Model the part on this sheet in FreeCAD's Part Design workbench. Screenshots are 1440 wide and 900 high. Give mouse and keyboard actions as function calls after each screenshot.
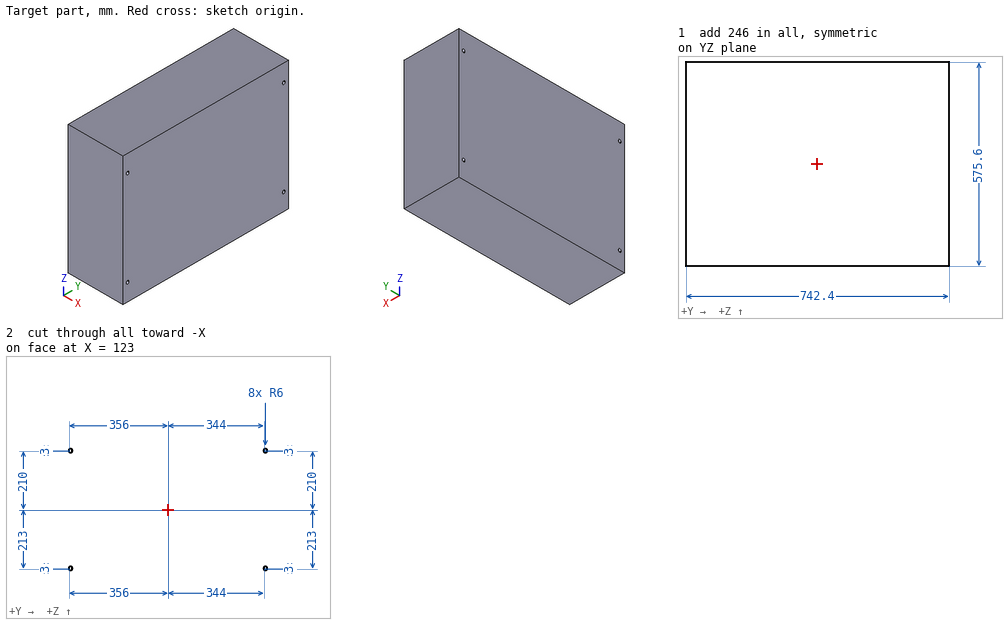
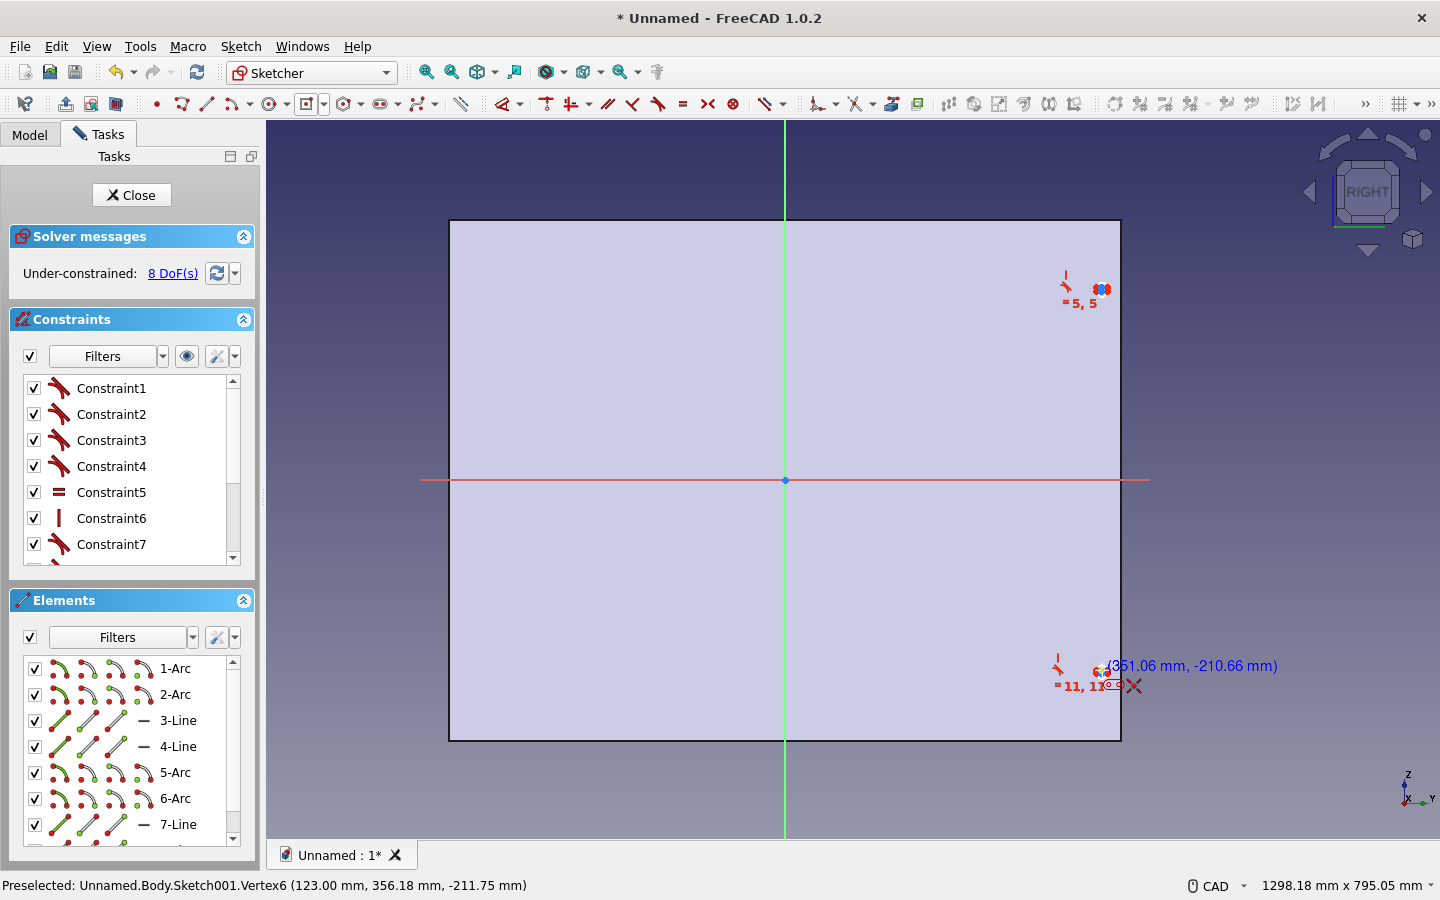
scroll(469, 673, up, 8)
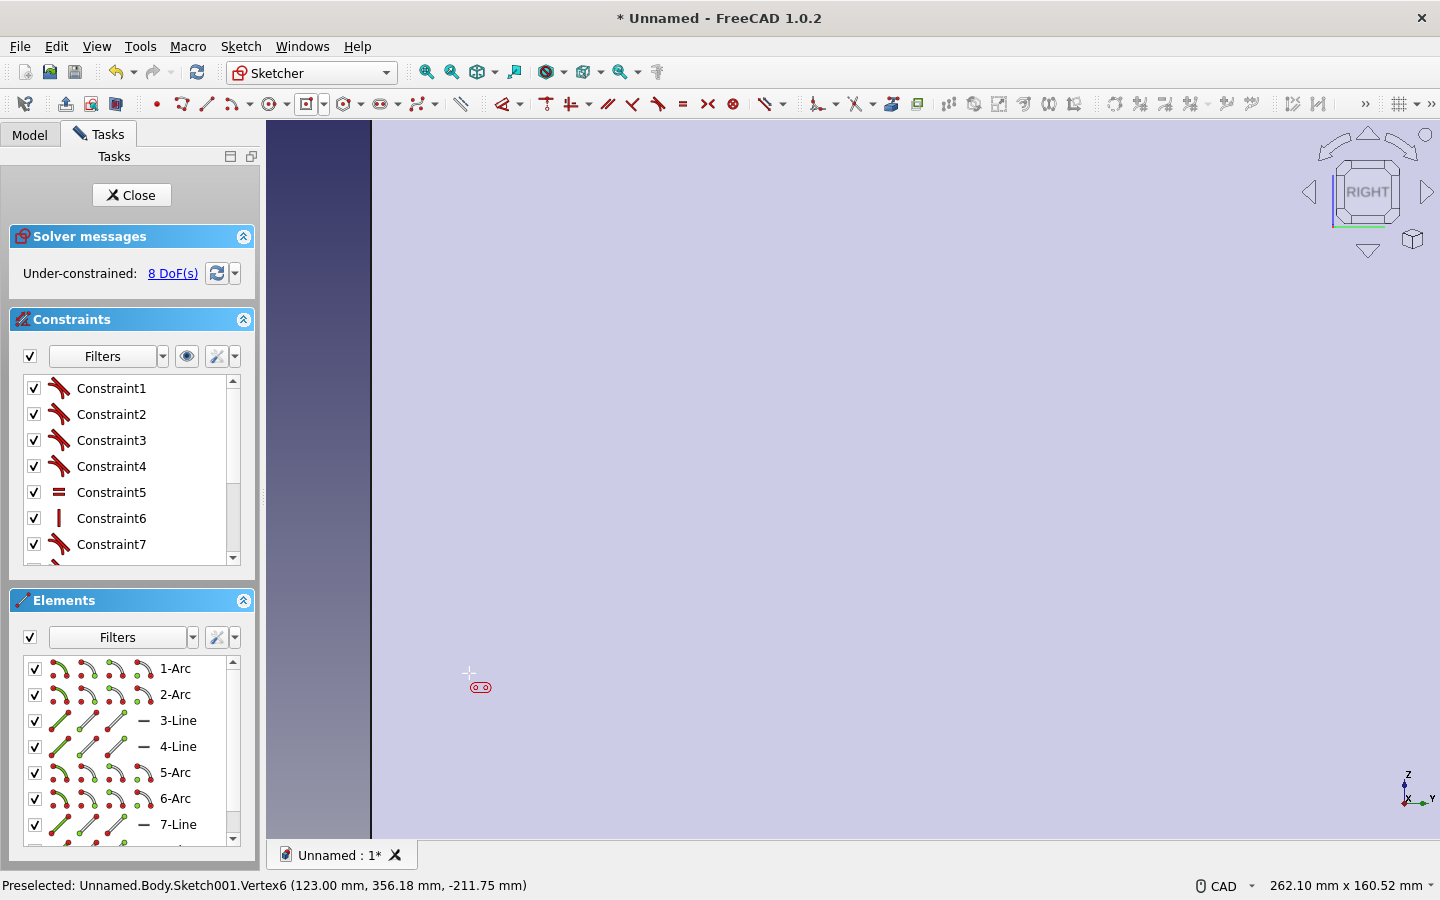
scroll(468, 673, down, 8)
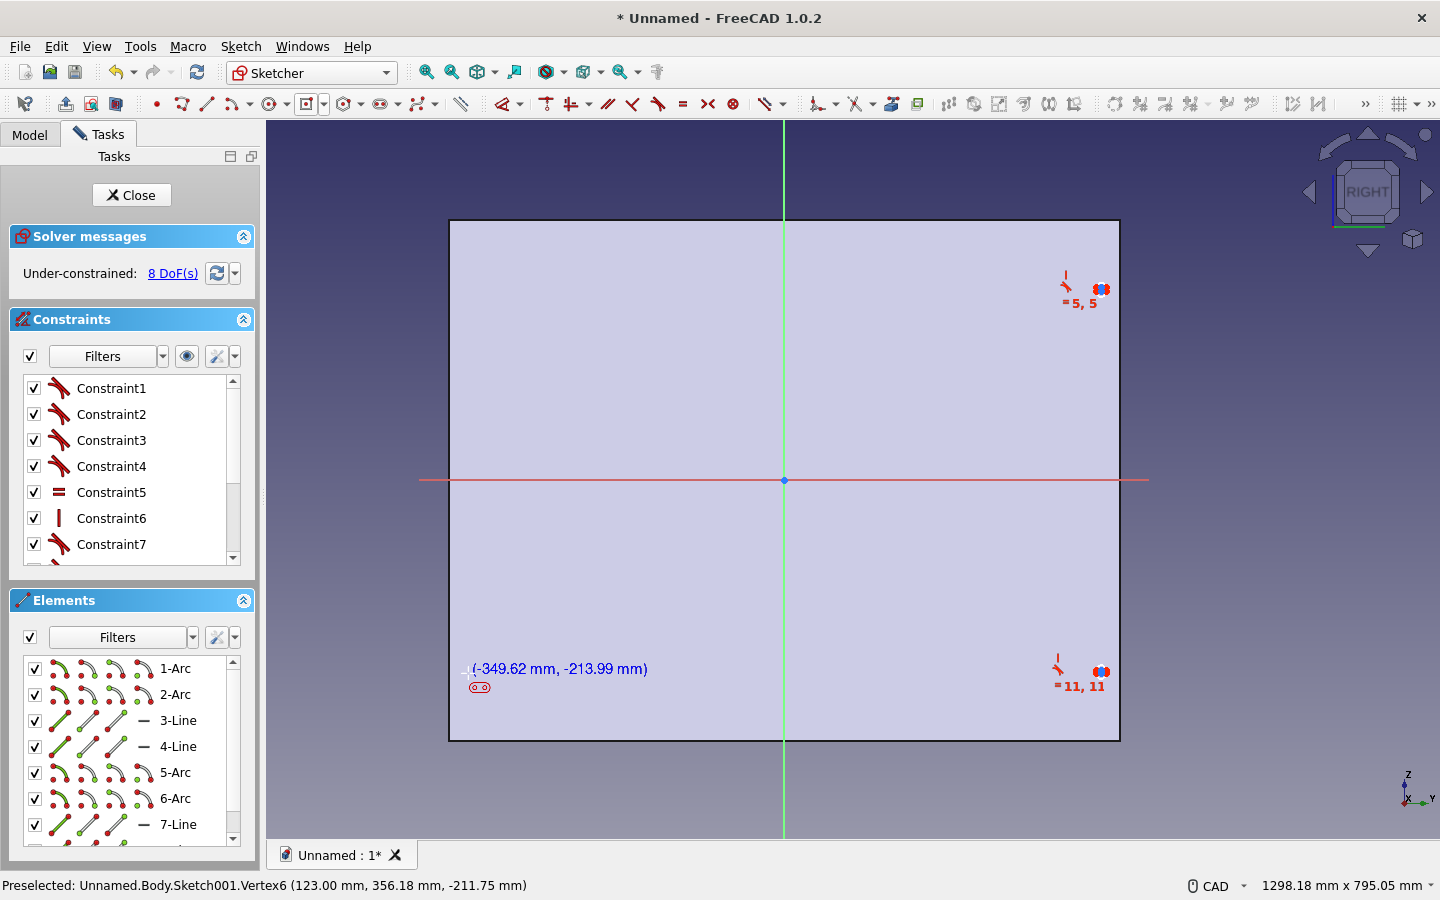
click(468, 673)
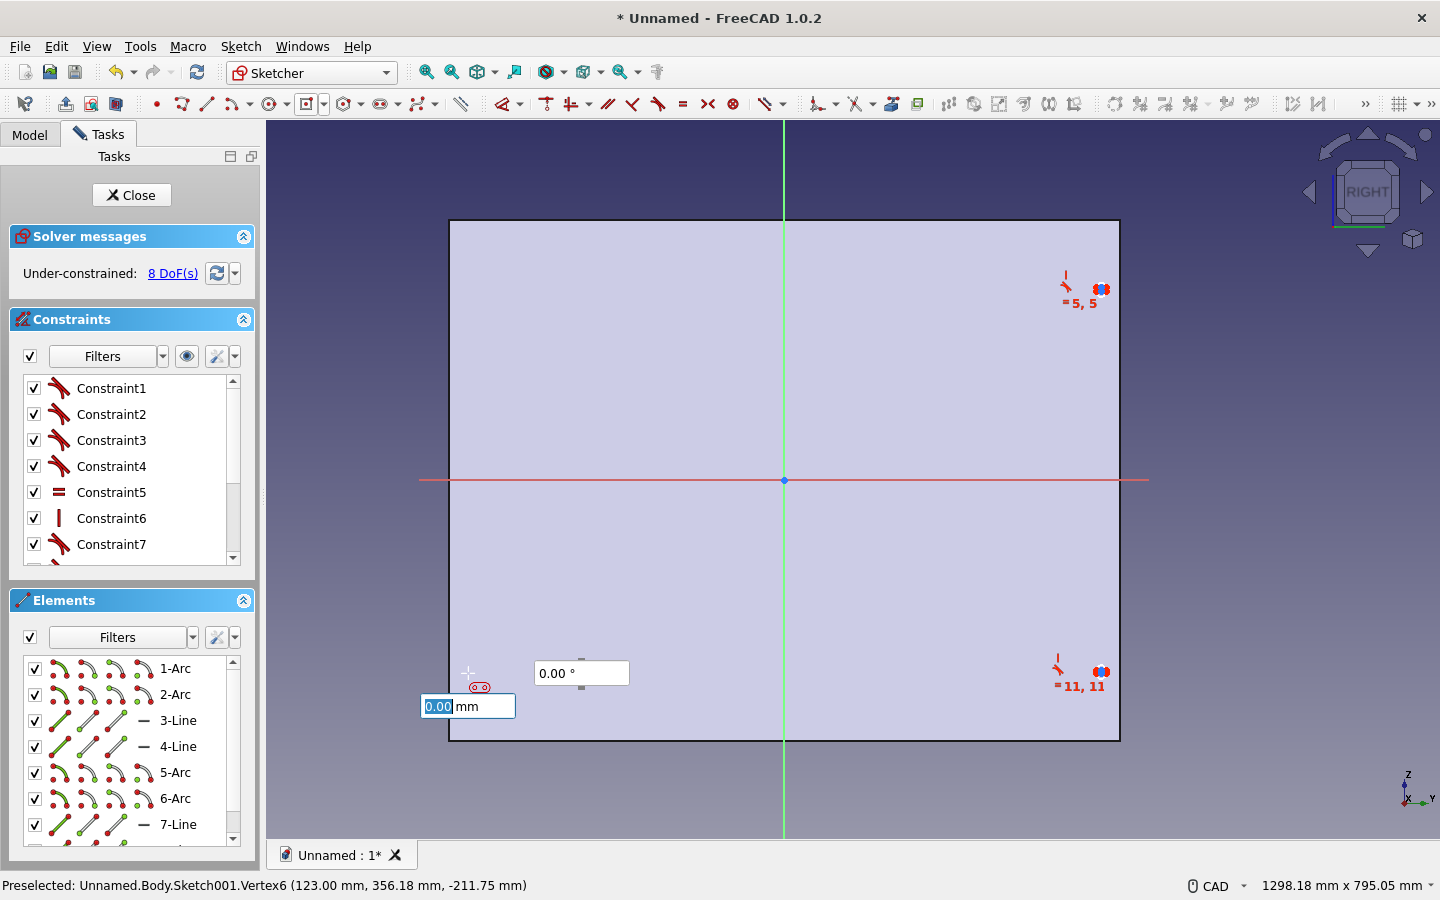
scroll(468, 670, up, 9)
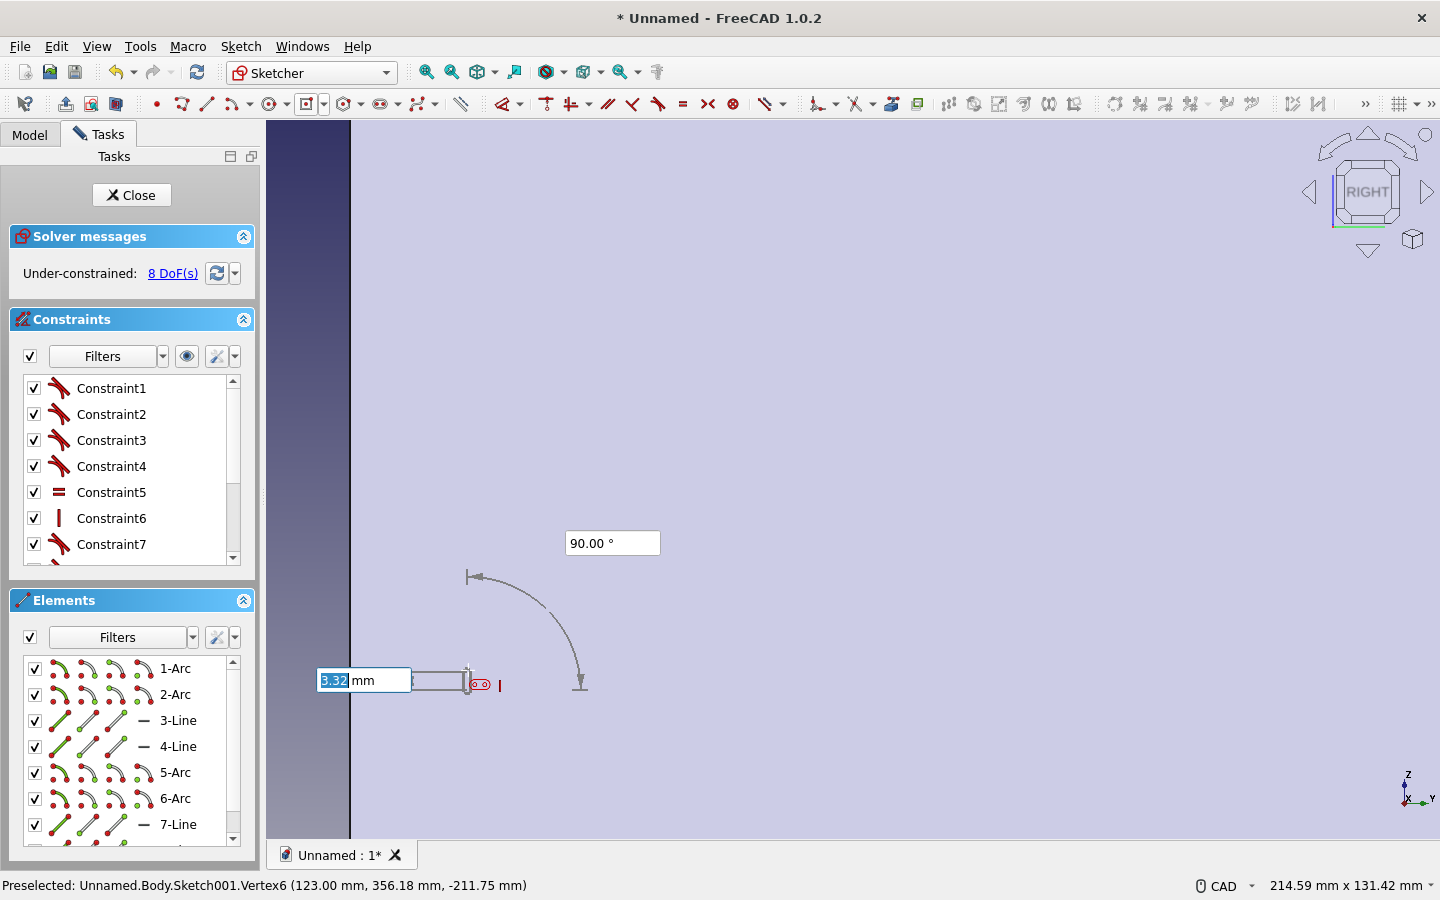
click(467, 667)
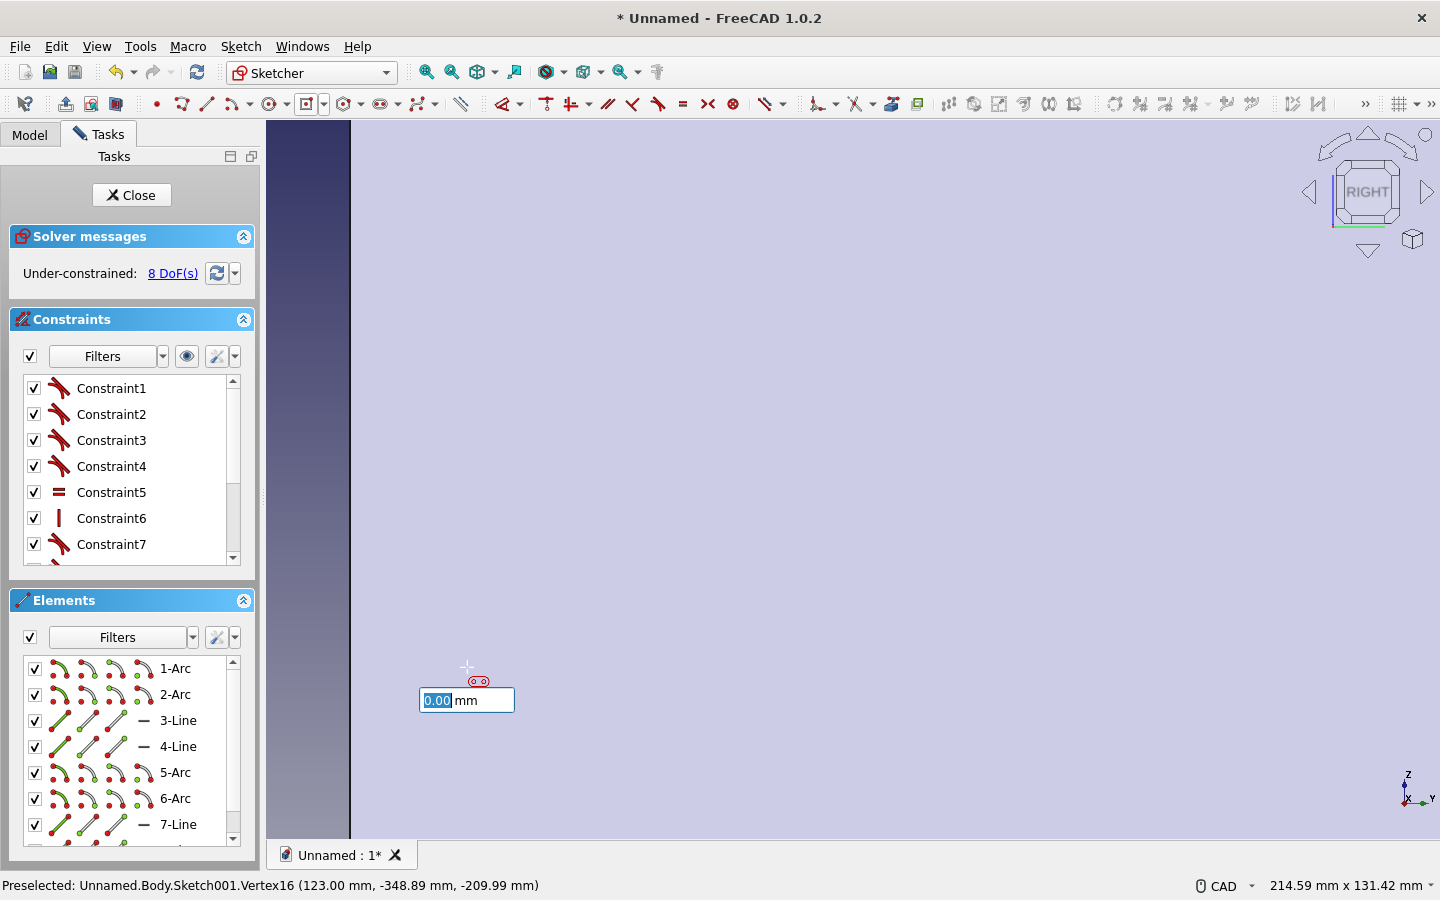
click(499, 676)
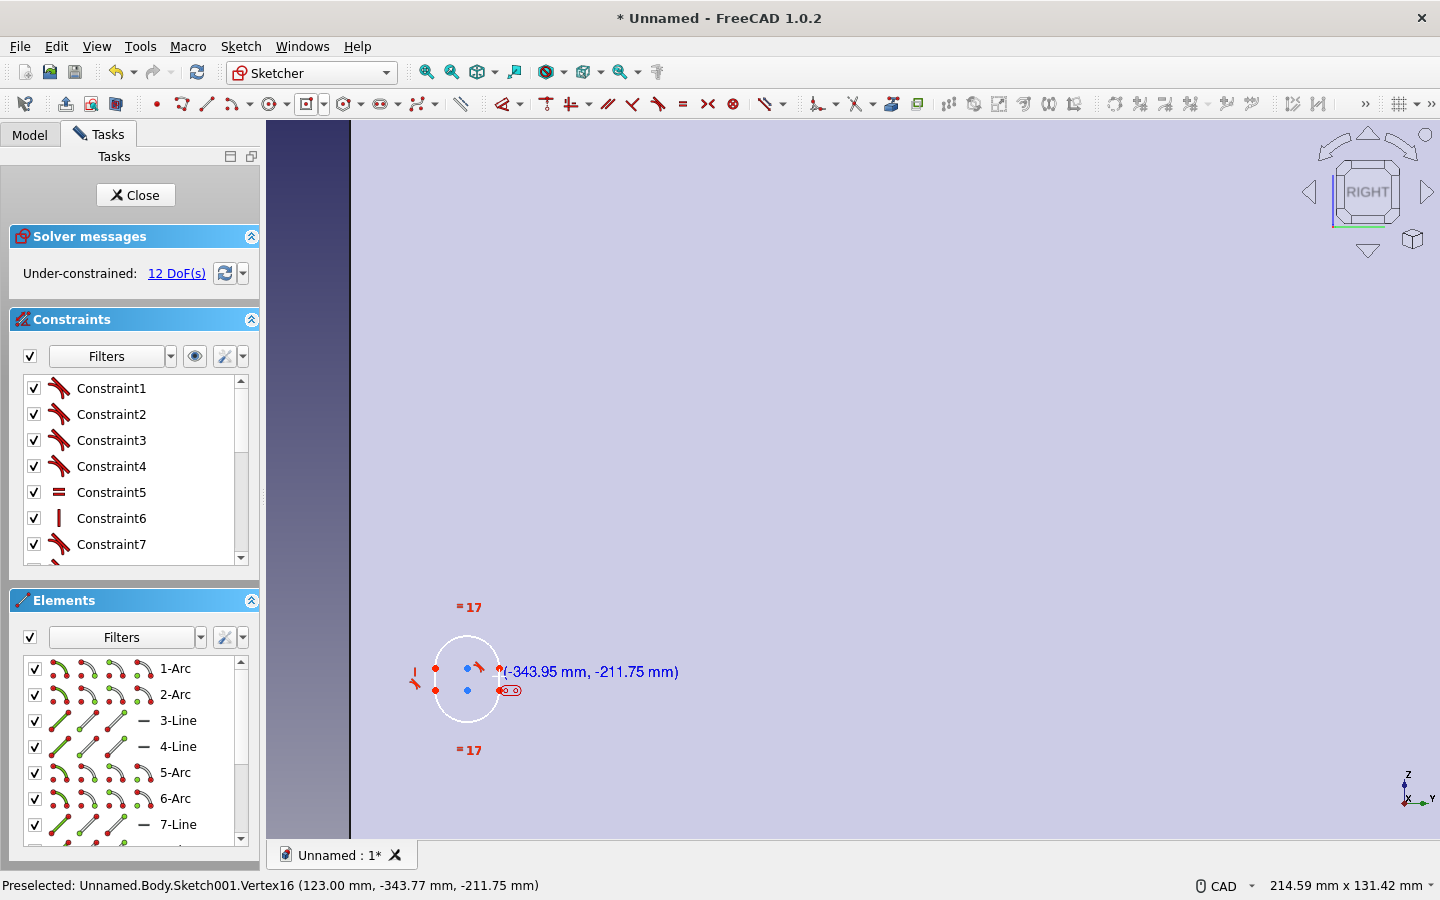
scroll(468, 670, down, 9)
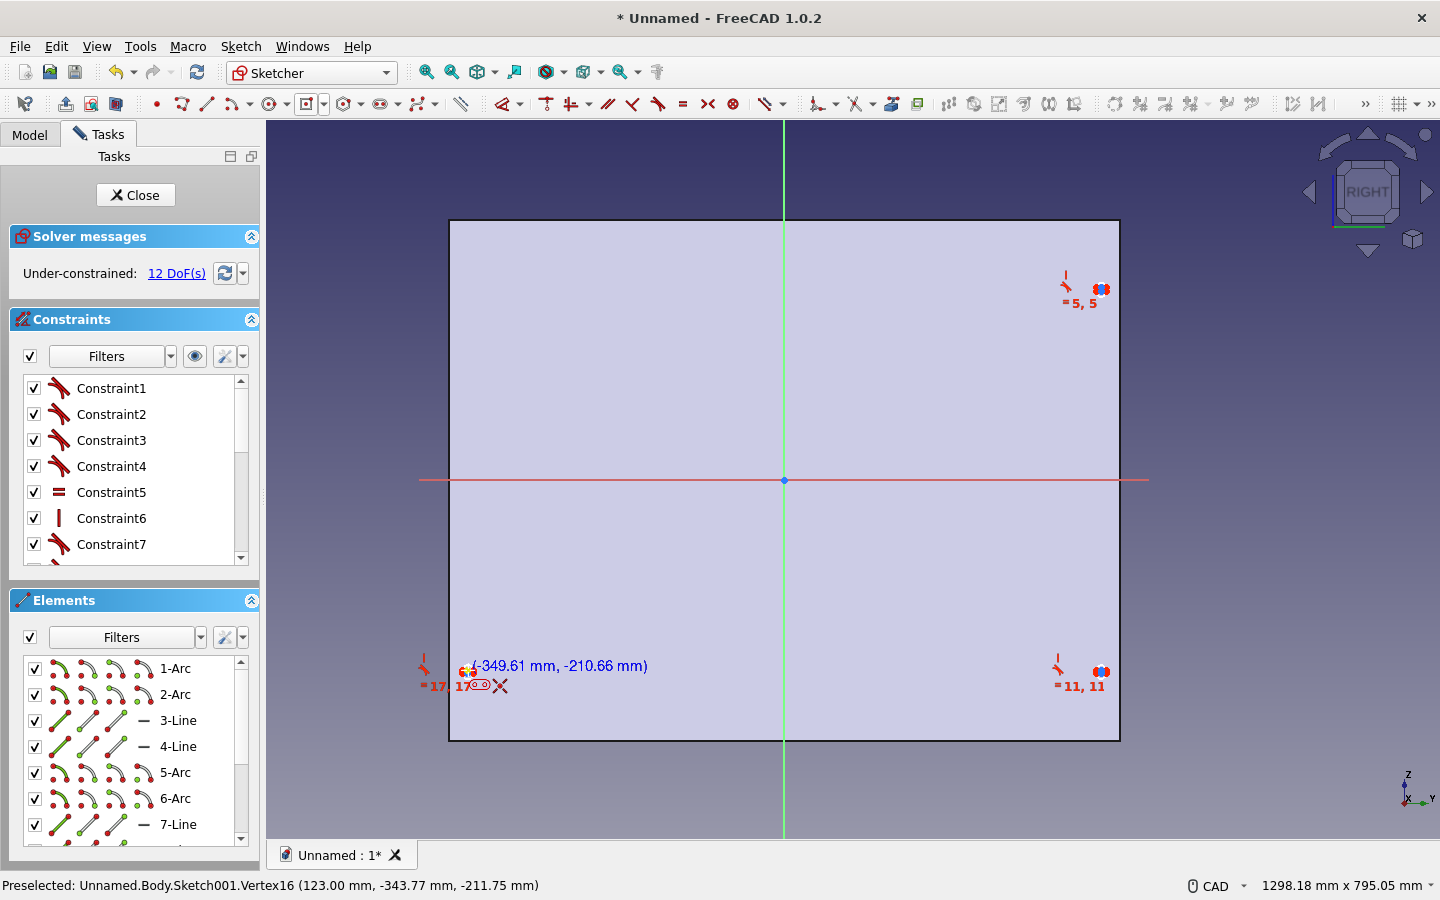
scroll(468, 290, up, 8)